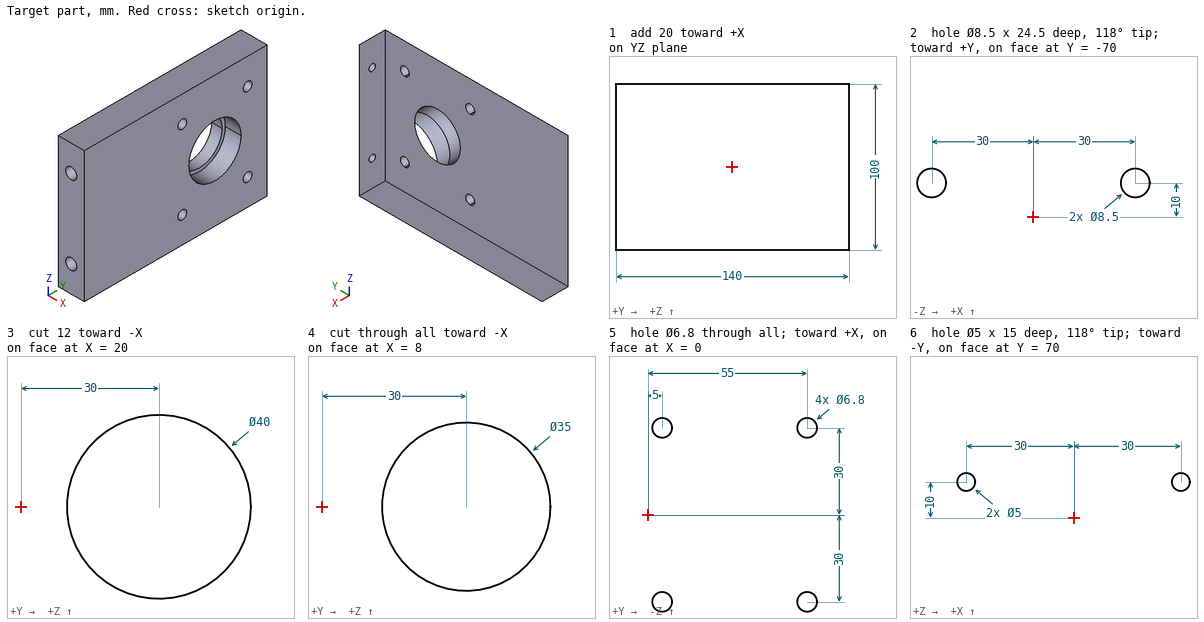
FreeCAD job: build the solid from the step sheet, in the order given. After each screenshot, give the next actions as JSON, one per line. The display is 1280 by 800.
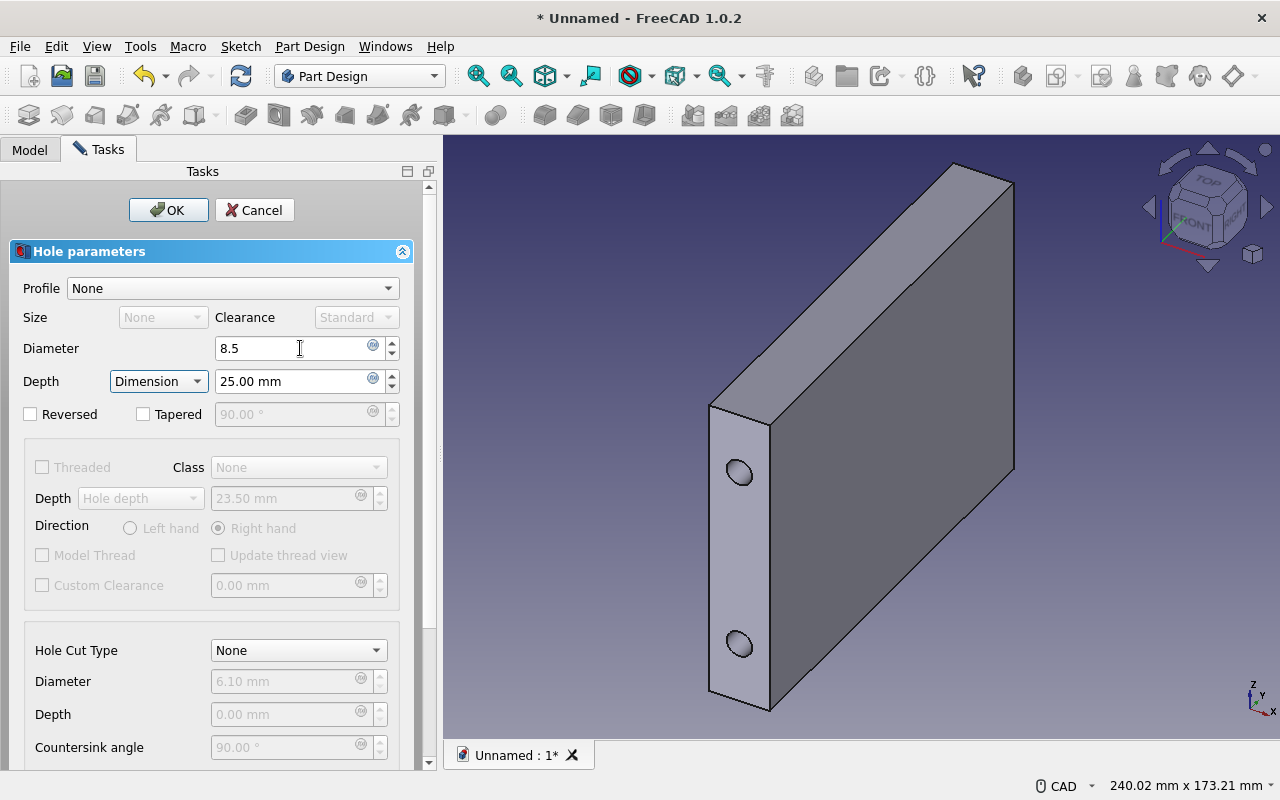
{"action": "triple_click", "coordinate": [300, 382]}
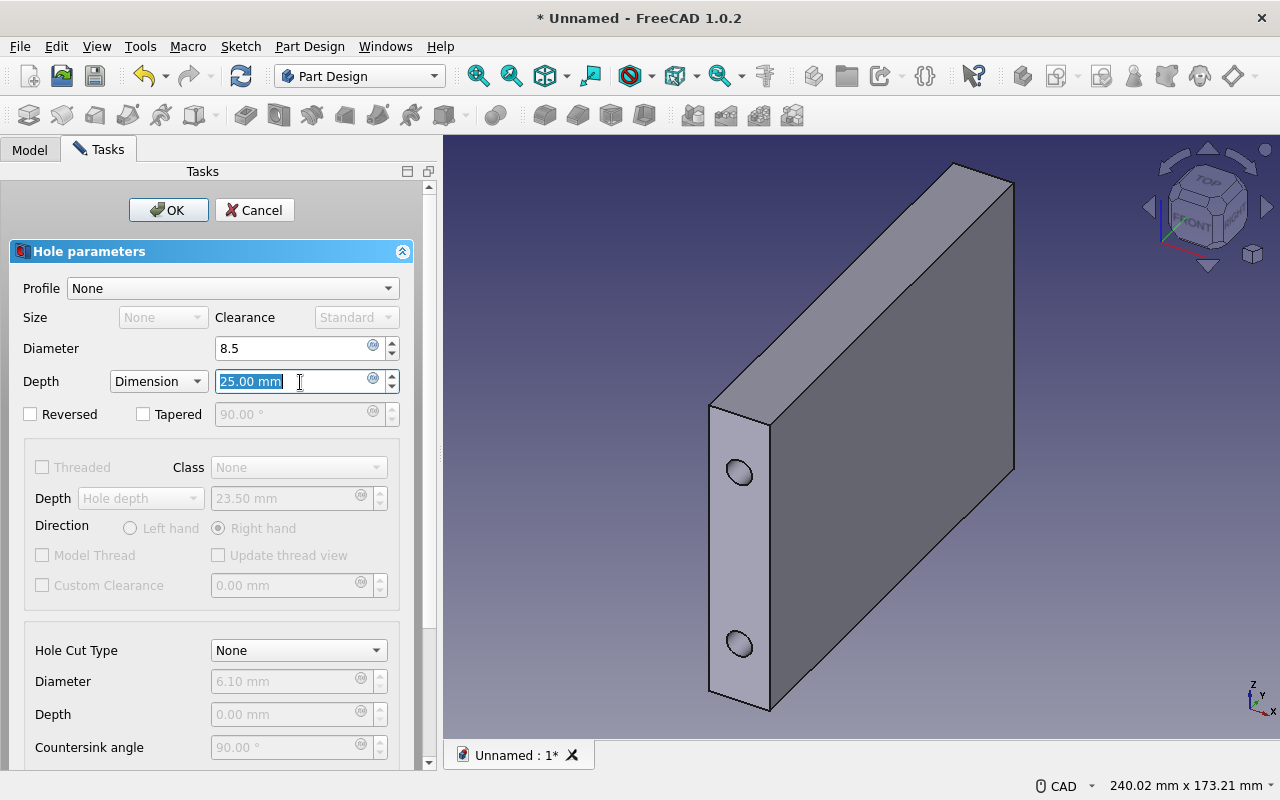
{"action": "type", "text": "24.5"}
{"action": "key", "text": "Tab"}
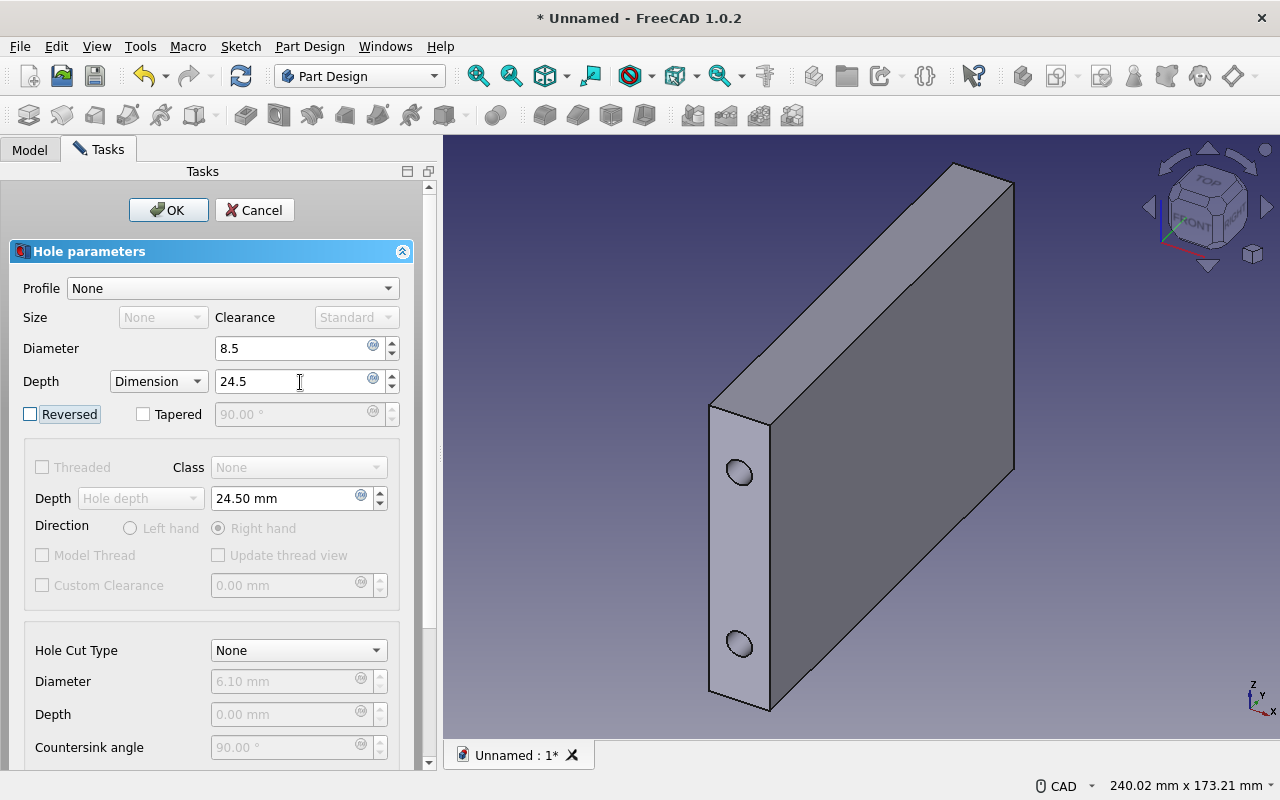
{"action": "left_click", "coordinate": [169, 210]}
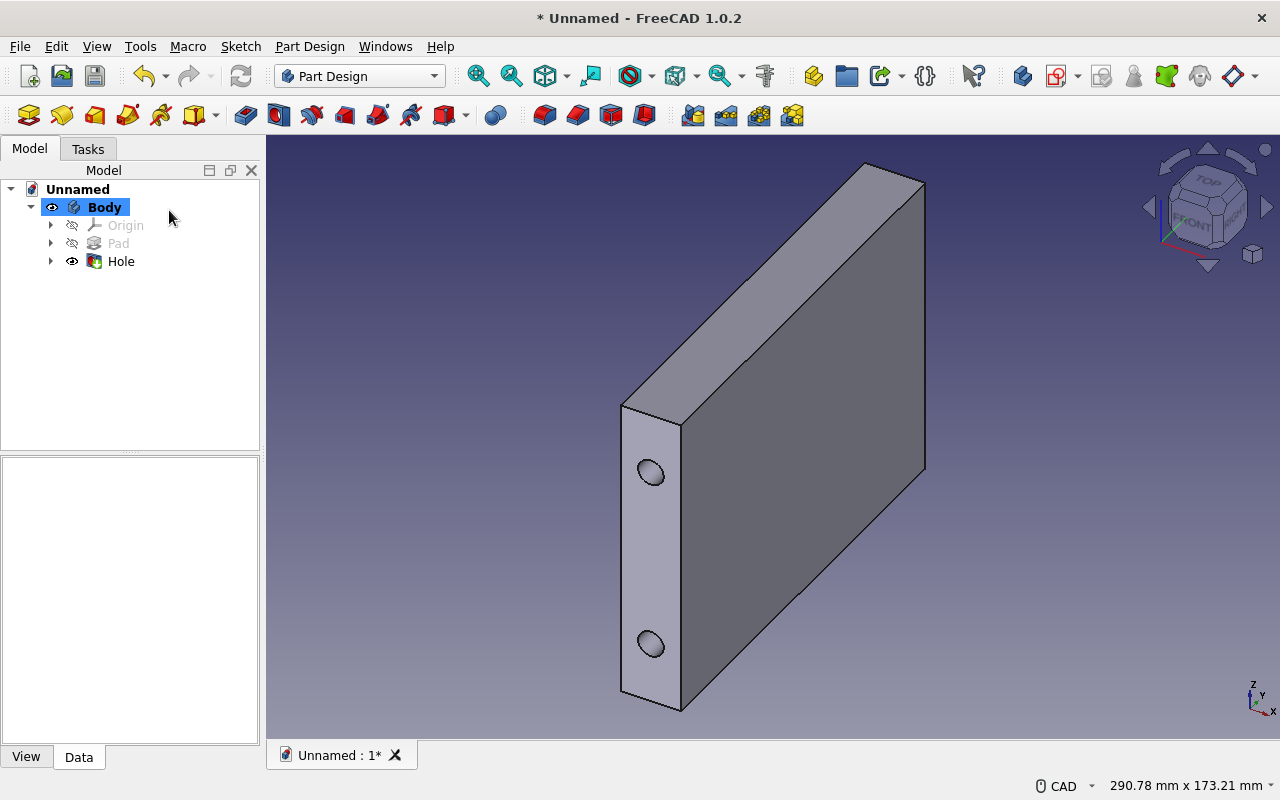
{"action": "left_click", "coordinate": [803, 446]}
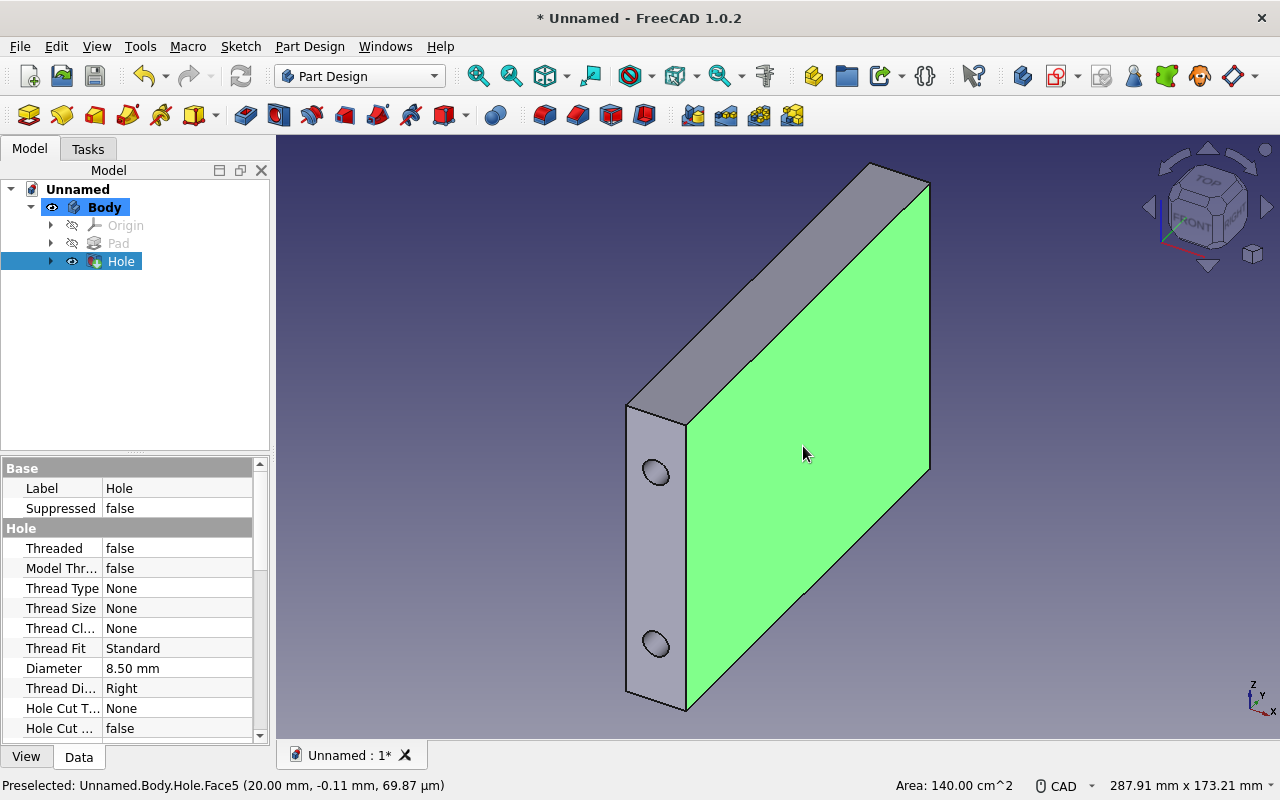
{"action": "left_click", "coordinate": [1056, 76]}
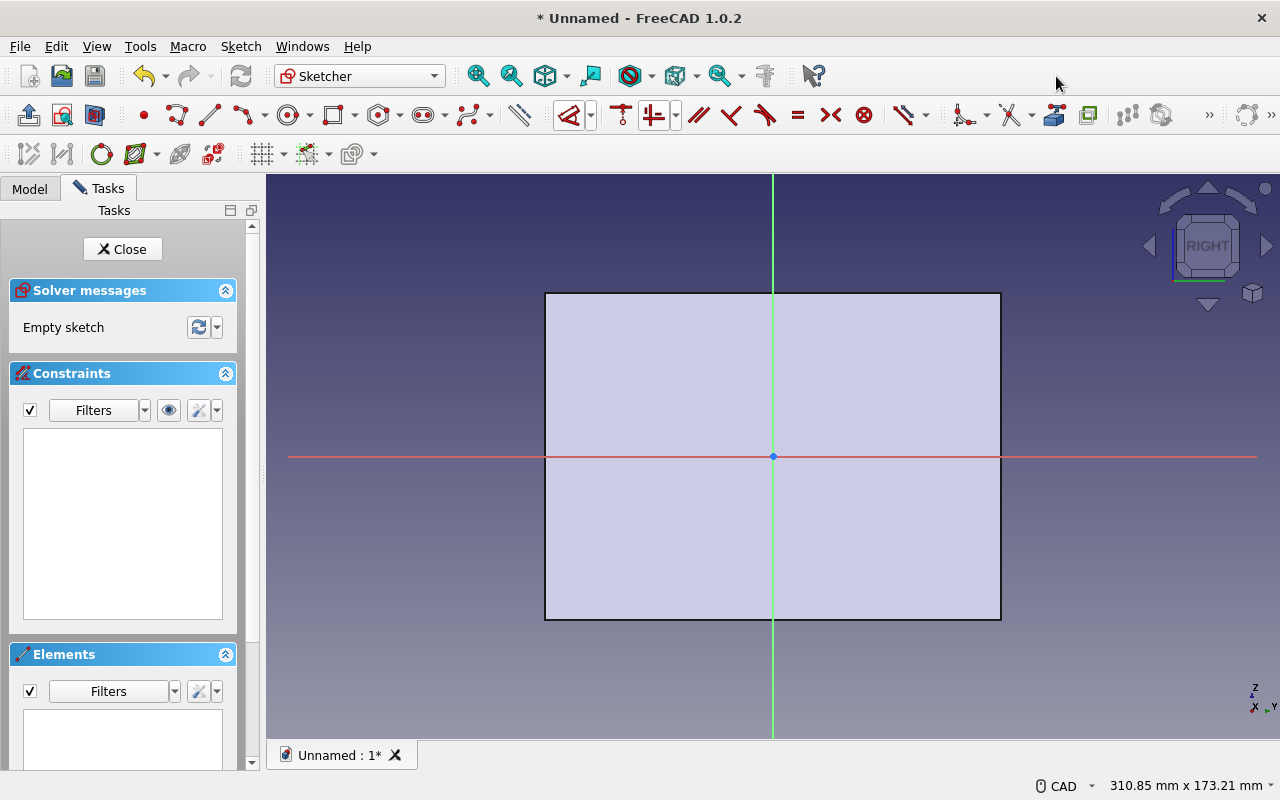
{"action": "scroll", "coordinate": [942, 456], "scroll_direction": "up", "scroll_amount": 5}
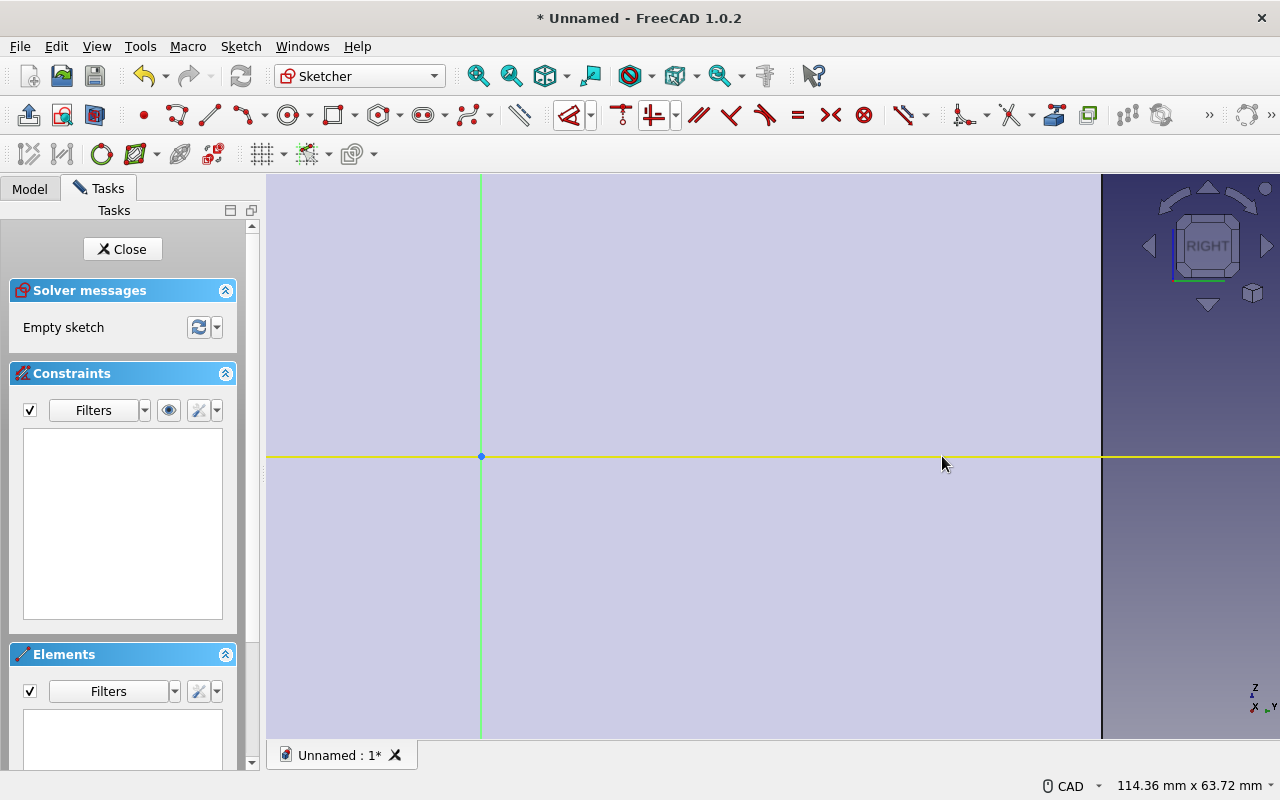
{"action": "left_click", "coordinate": [288, 116]}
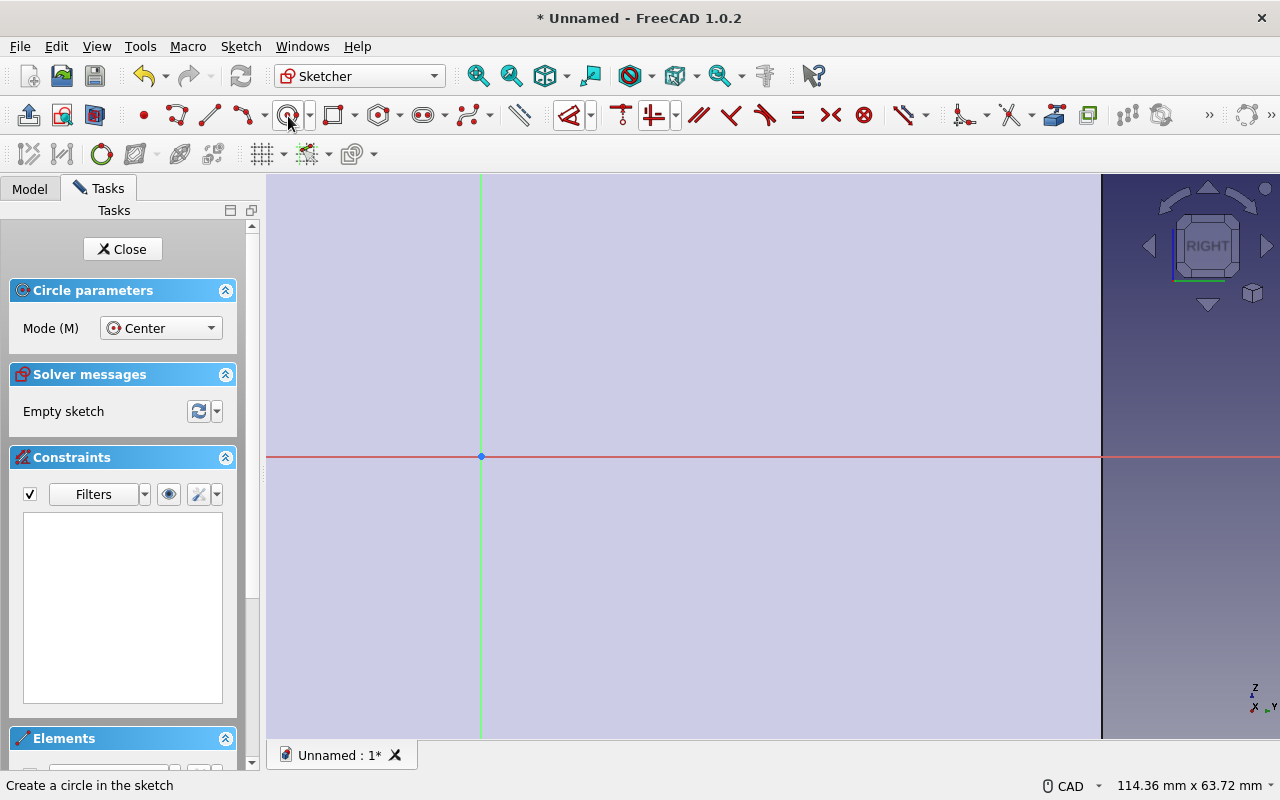
{"action": "left_click", "coordinate": [747, 456]}
{"action": "mouse_move", "coordinate": [873, 331]}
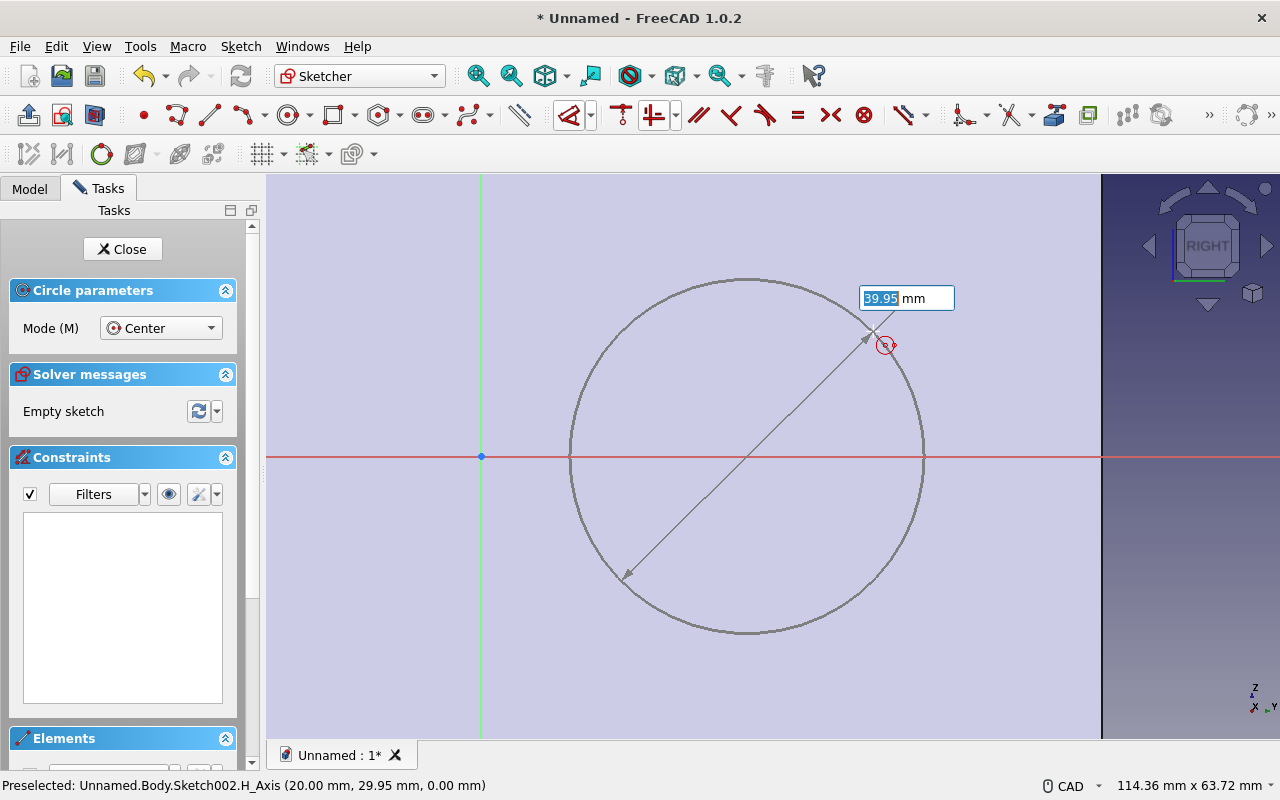
{"action": "type", "text": "40"}
{"action": "key", "text": "Return"}
{"action": "key", "text": "Escape"}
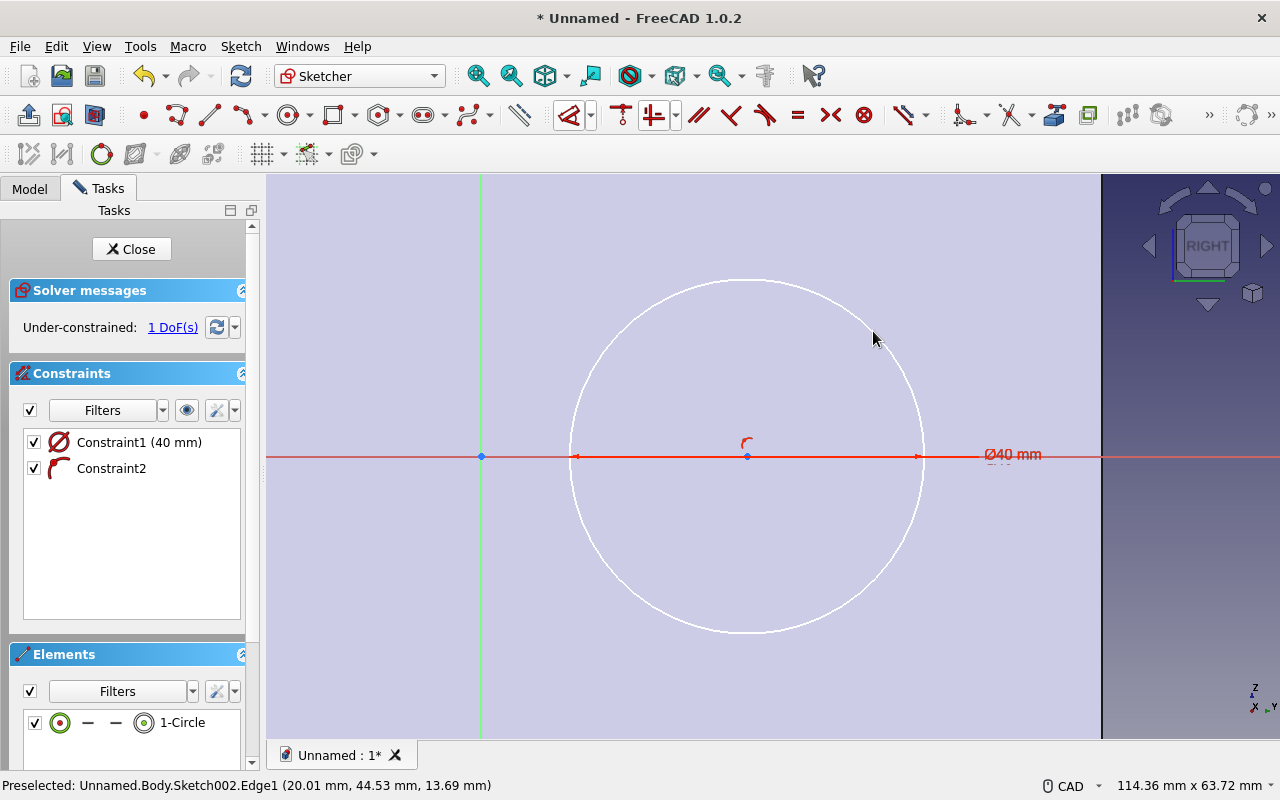
{"action": "left_click", "coordinate": [747, 456]}